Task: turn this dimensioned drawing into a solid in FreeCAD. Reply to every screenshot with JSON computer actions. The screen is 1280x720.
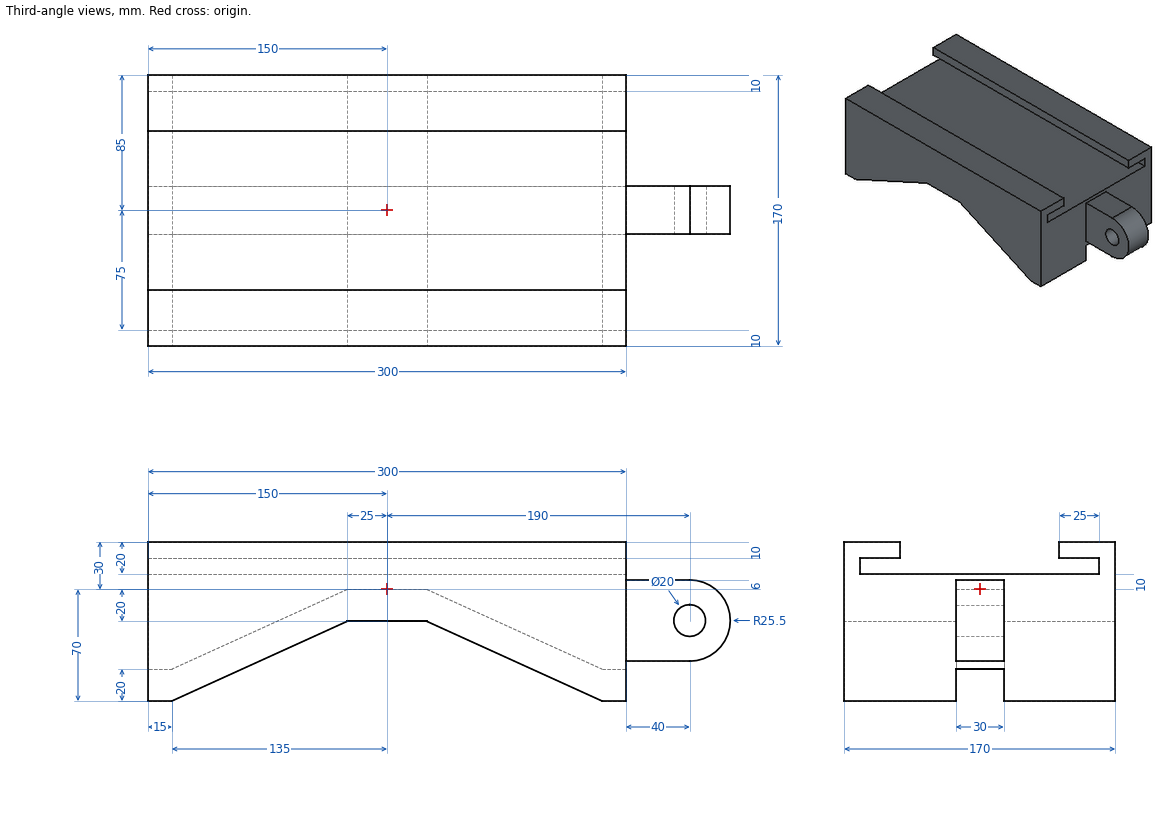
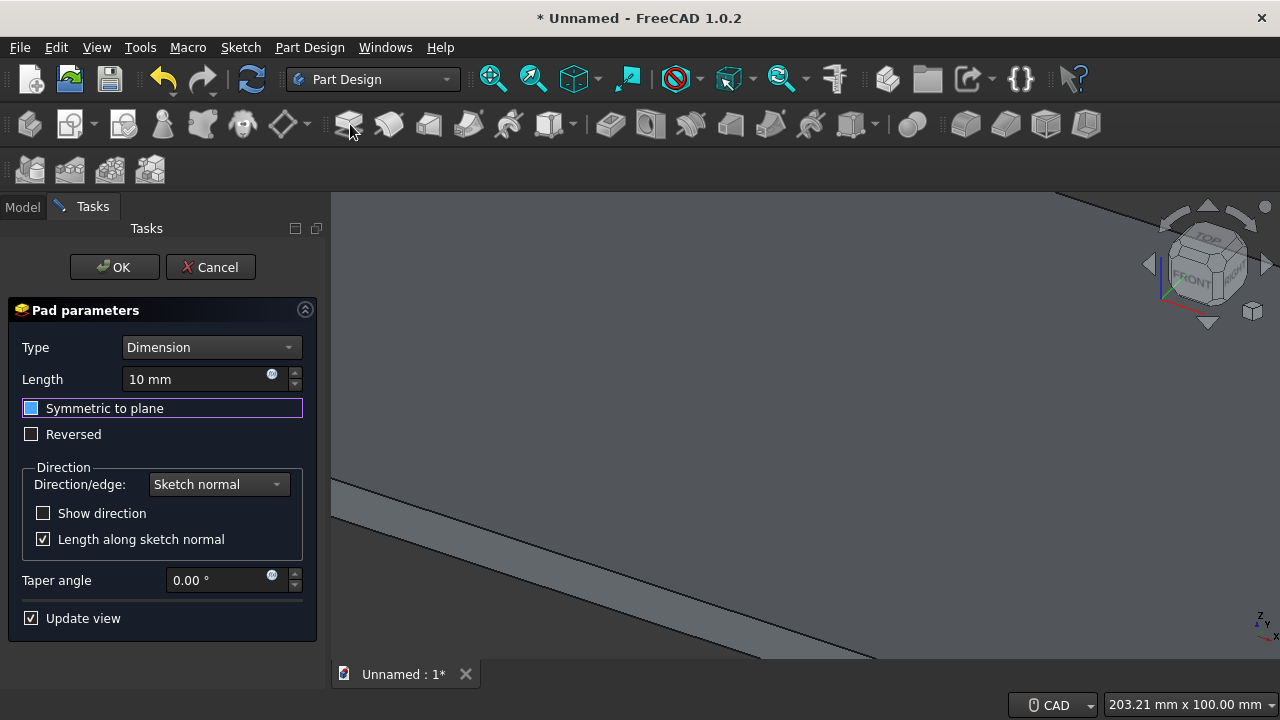
{"action": "left_click", "coordinate": [115, 267]}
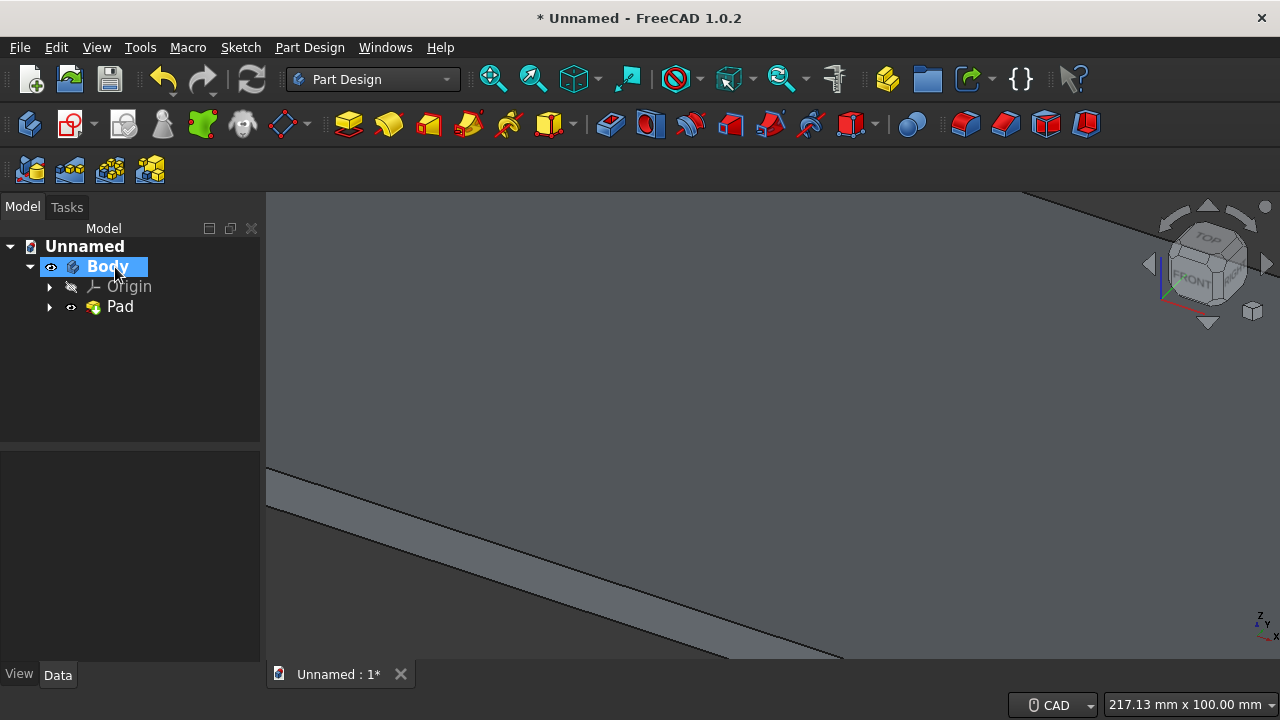
{"action": "key", "text": "v f"}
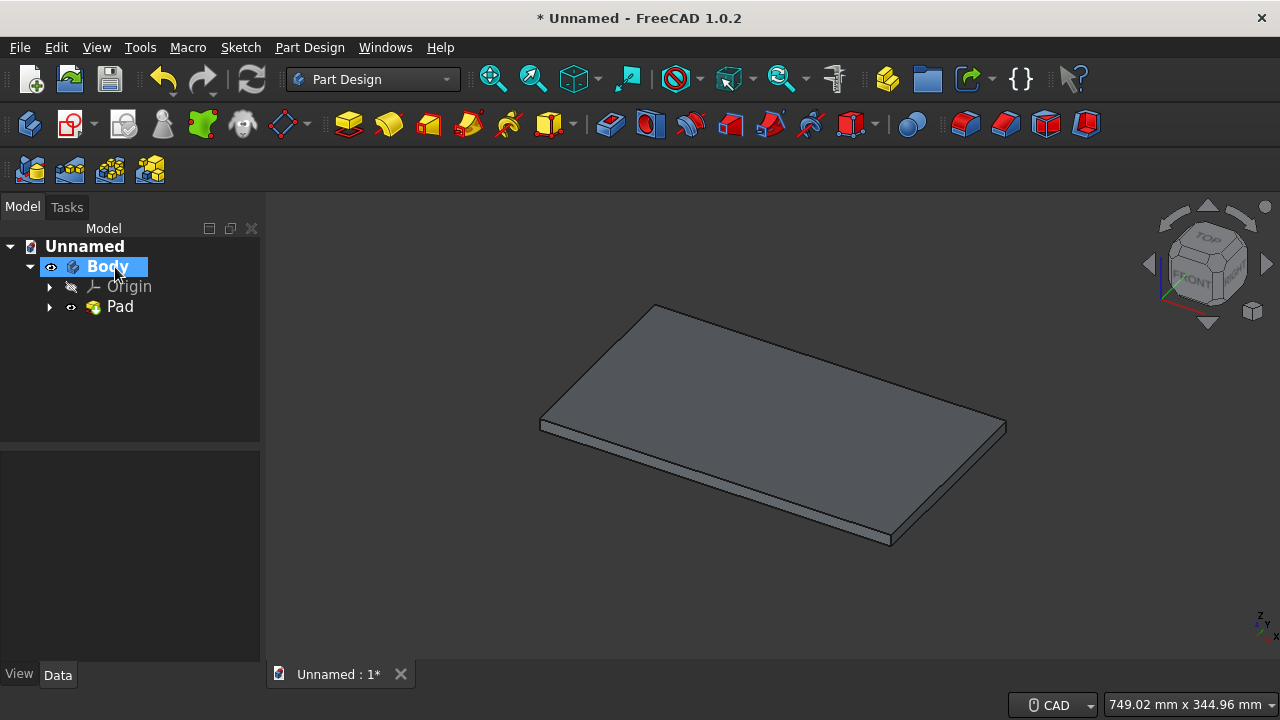
{"action": "left_click", "coordinate": [823, 436]}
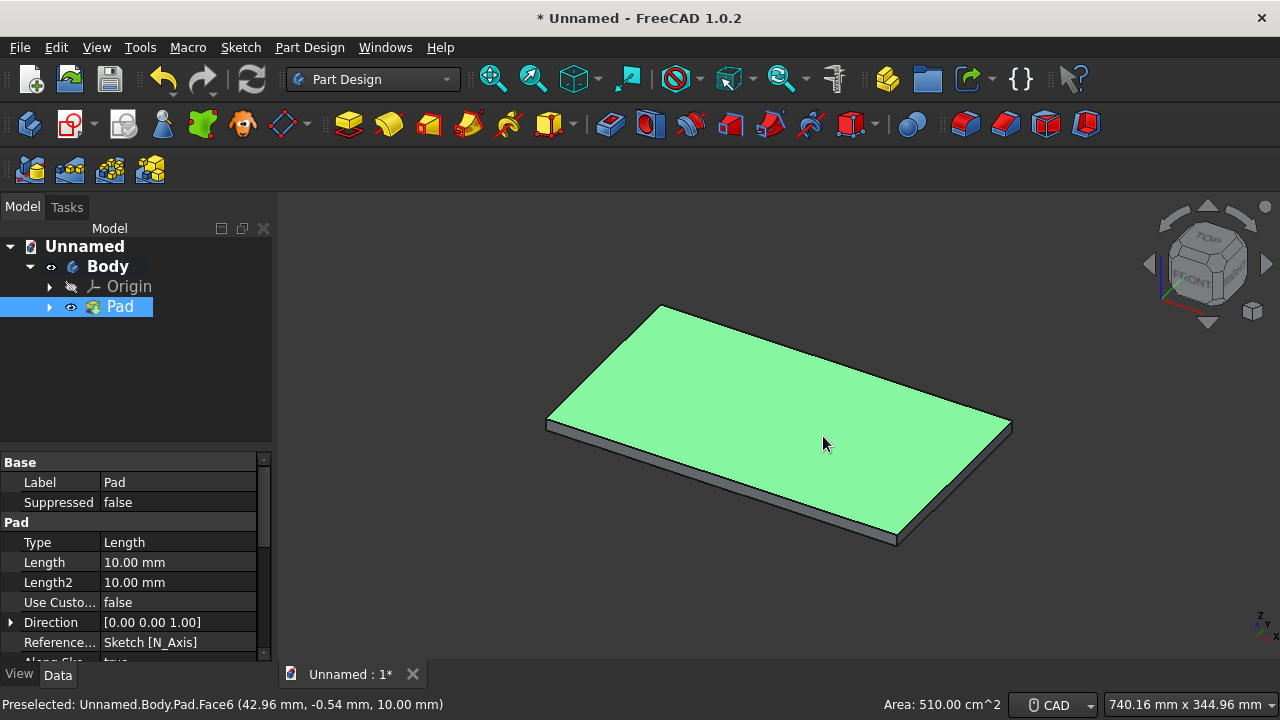
{"action": "left_click", "coordinate": [70, 124]}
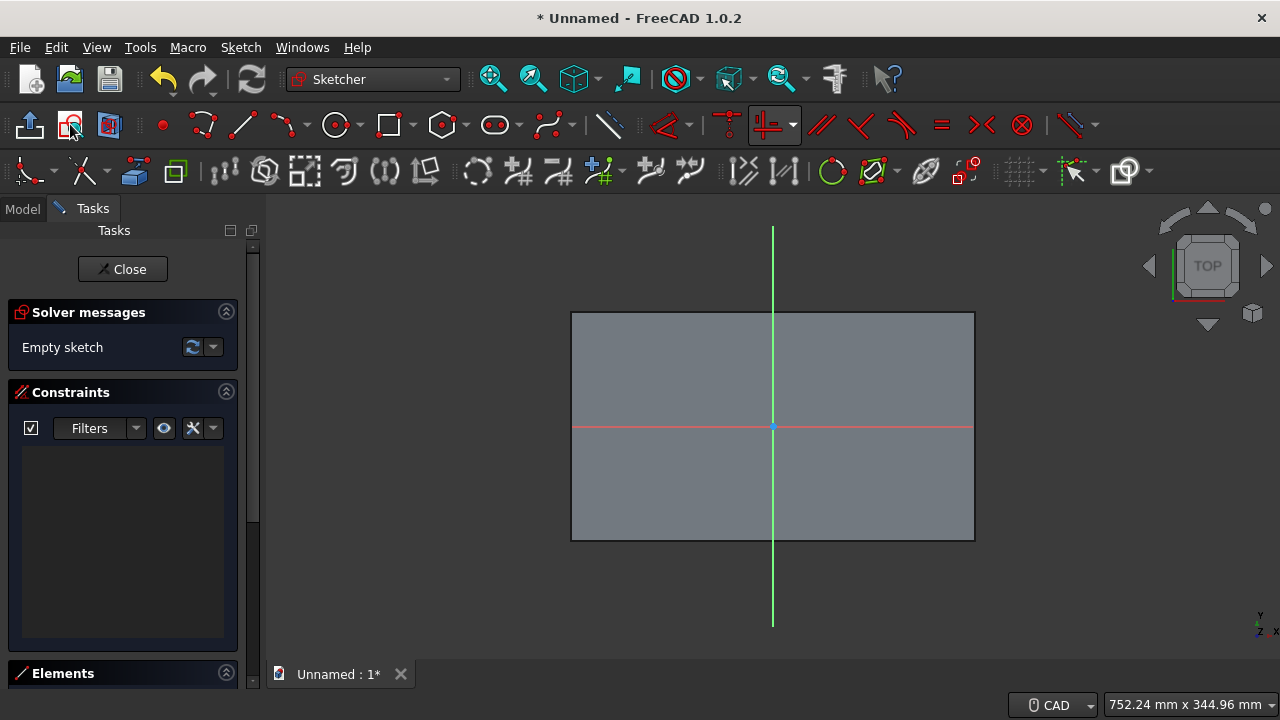
{"action": "key", "text": "g r"}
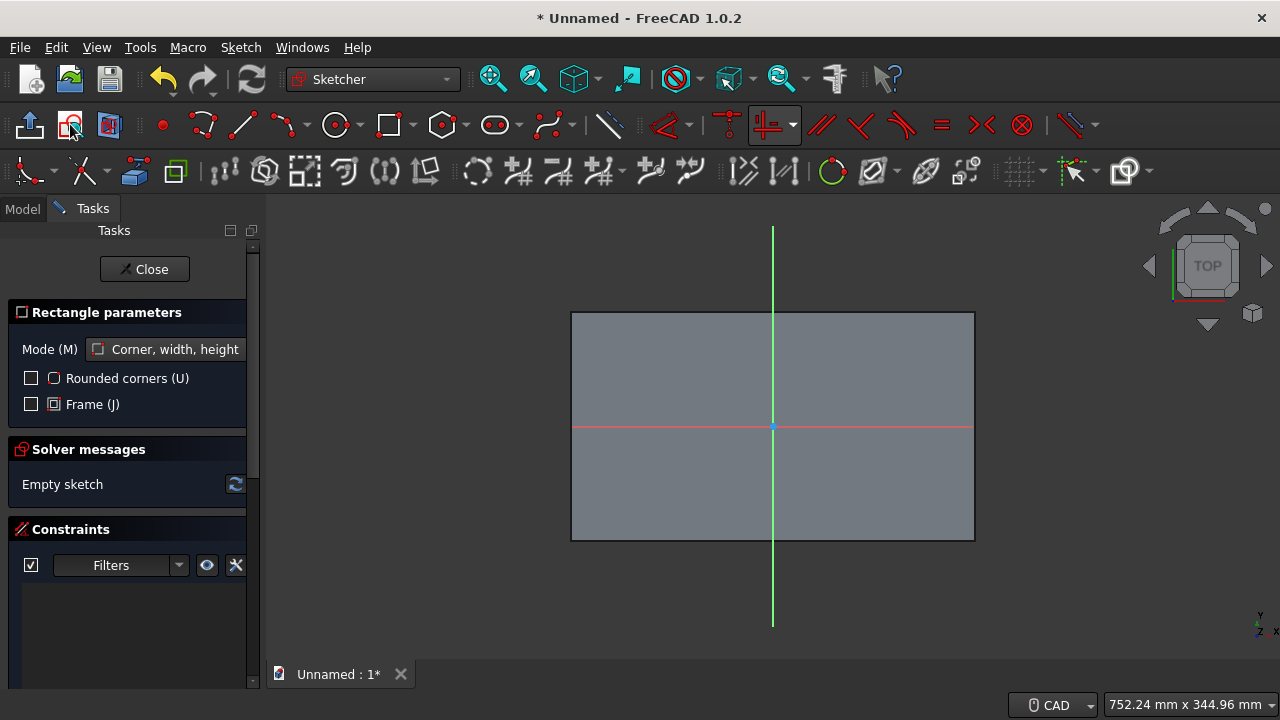
{"action": "left_click", "coordinate": [571, 312]}
{"action": "mouse_move", "coordinate": [975, 325]}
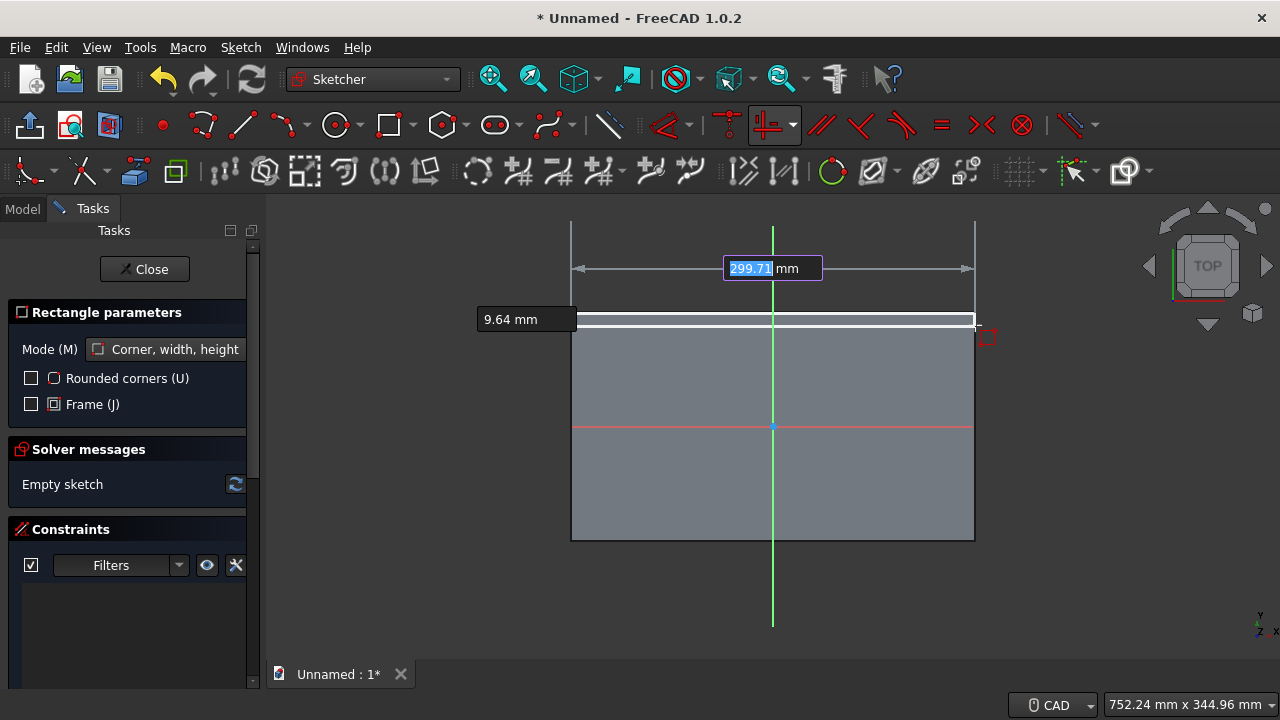
{"action": "type", "text": "300"}
{"action": "key", "text": "Tab"}
{"action": "type", "text": "10"}
{"action": "key", "text": "Return"}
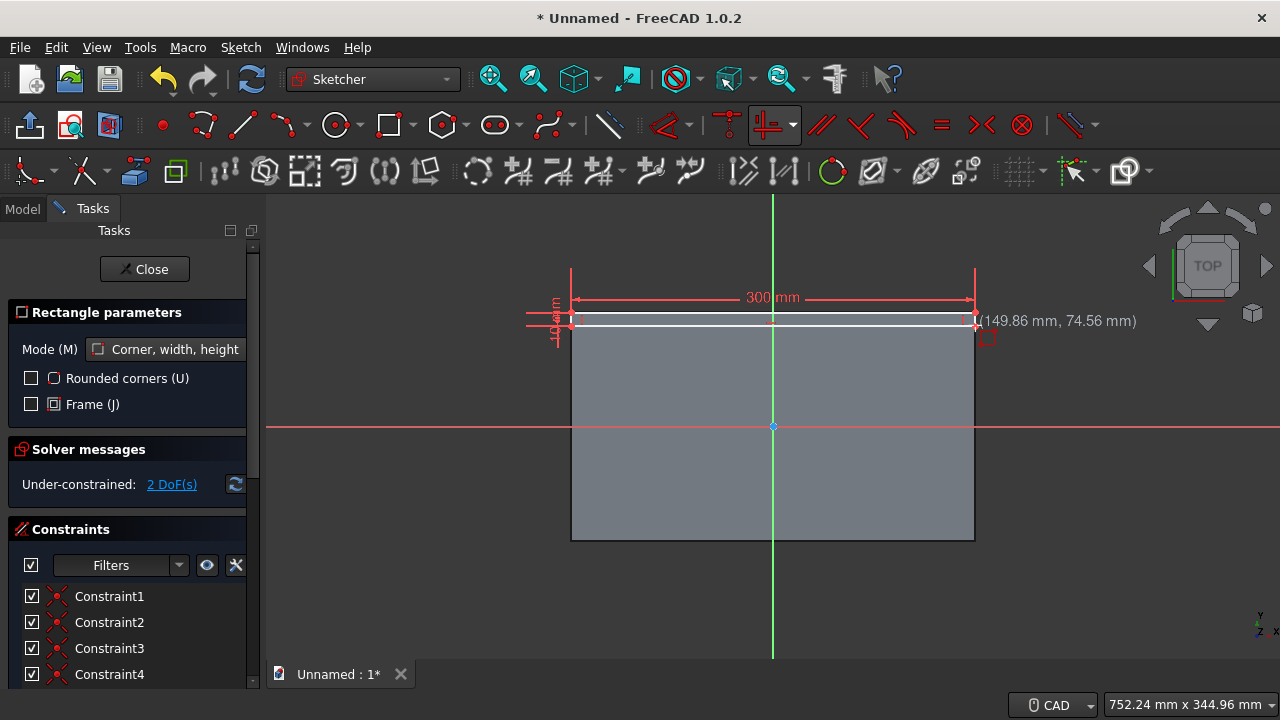
{"action": "left_click", "coordinate": [571, 528]}
{"action": "mouse_move", "coordinate": [975, 541]}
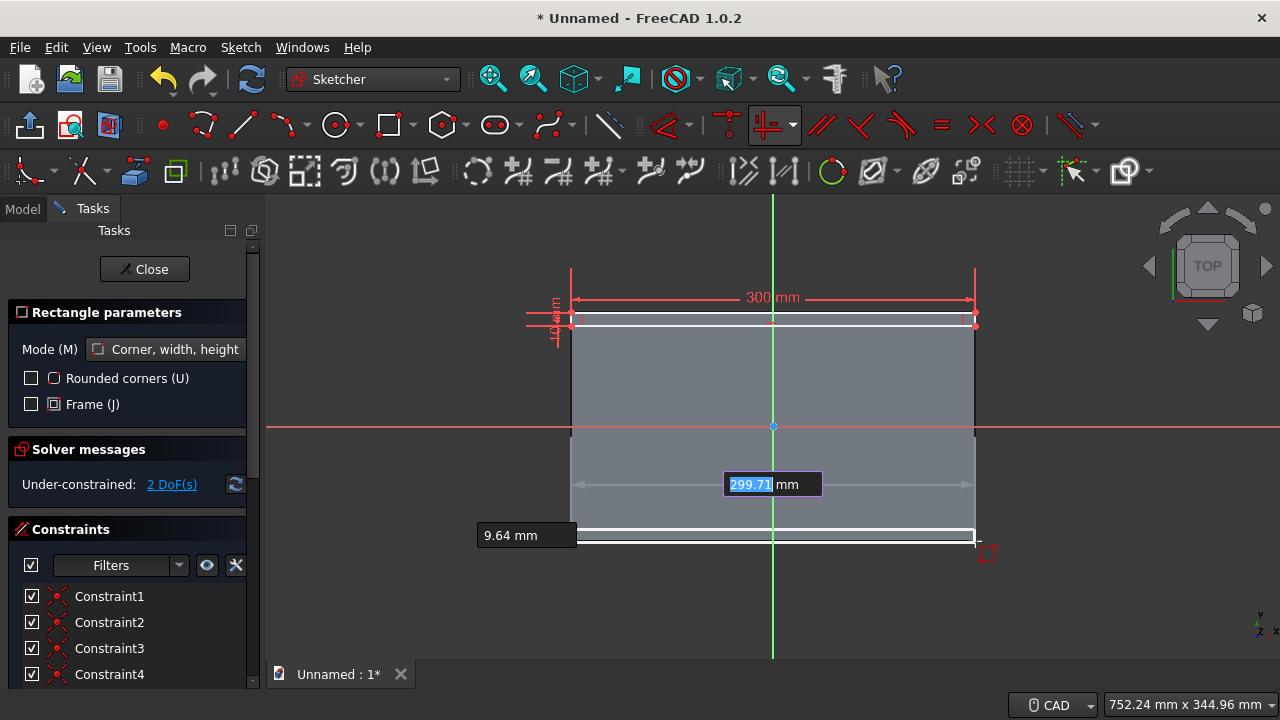
{"action": "type", "text": "300"}
{"action": "key", "text": "Tab"}
{"action": "type", "text": "10"}
{"action": "key", "text": "Return"}
{"action": "key", "text": "Escape"}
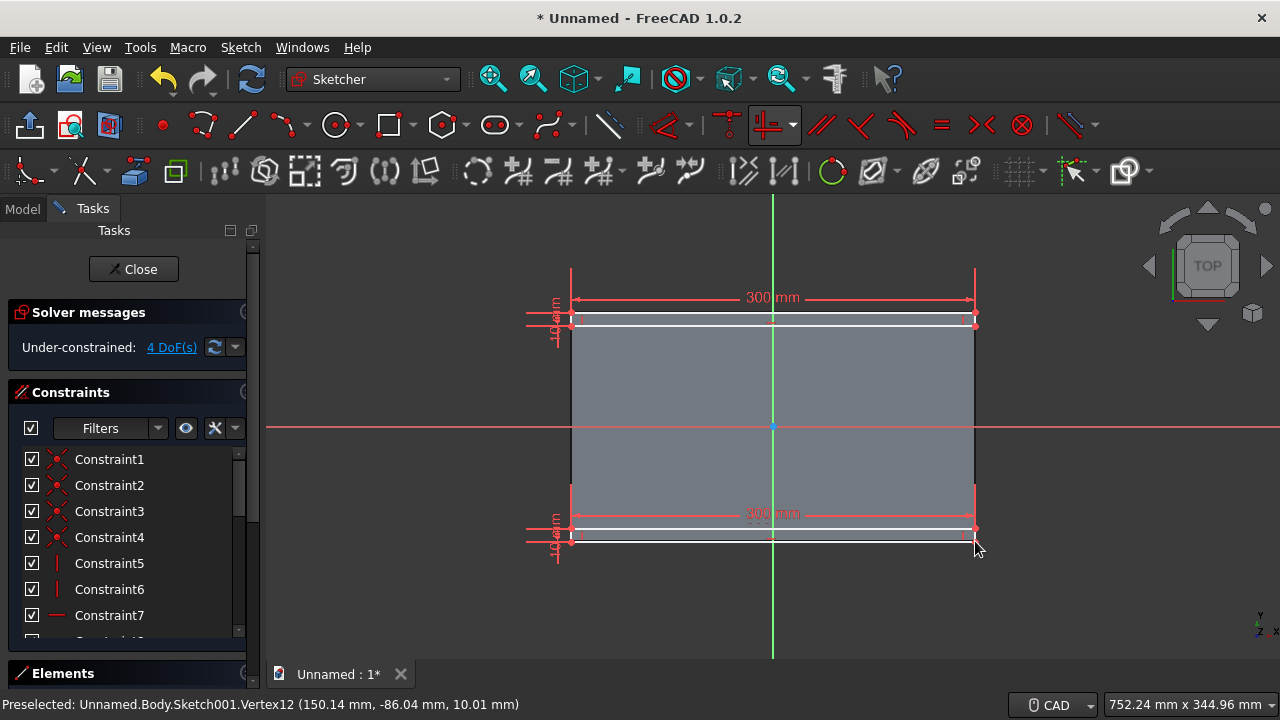
{"action": "left_click", "coordinate": [664, 126]}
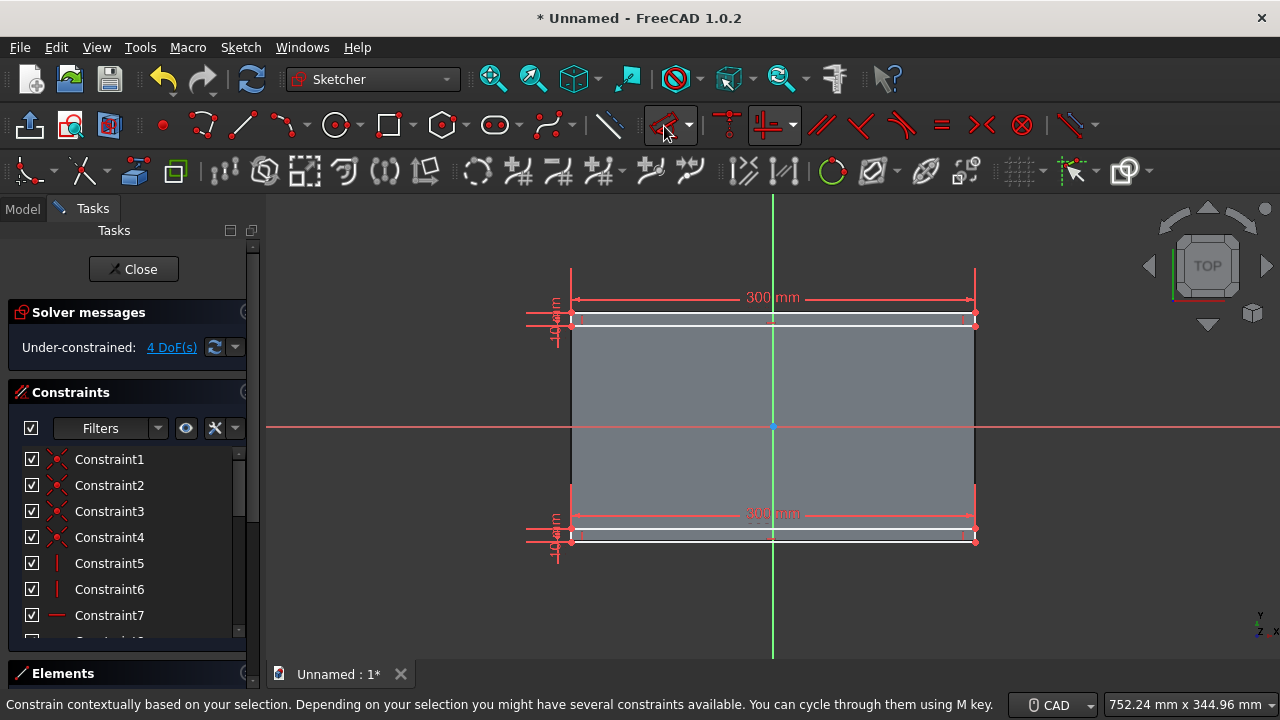
{"action": "left_click", "coordinate": [571, 313]}
{"action": "left_click", "coordinate": [537, 370]}